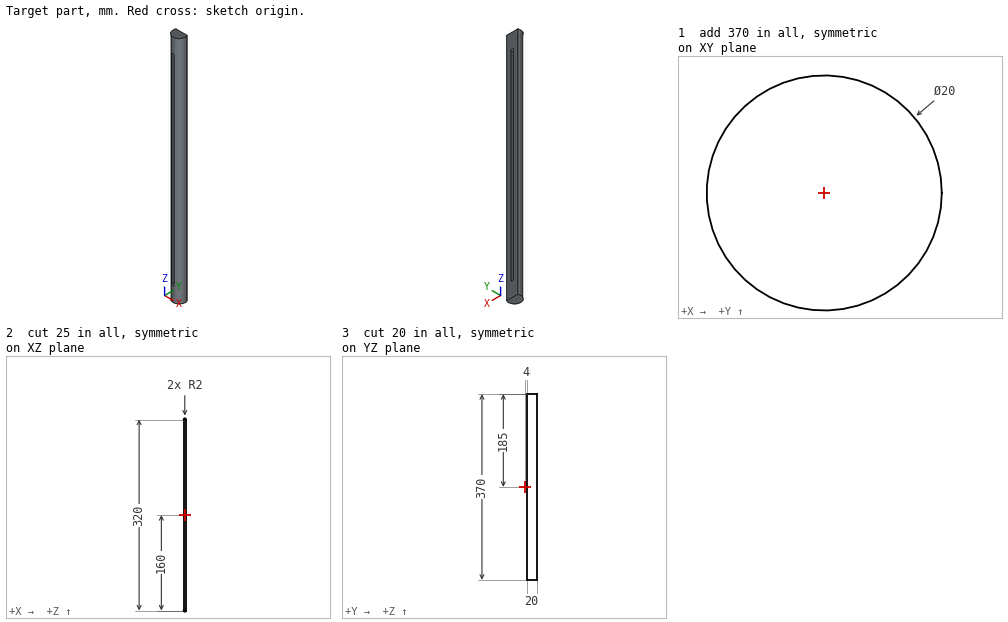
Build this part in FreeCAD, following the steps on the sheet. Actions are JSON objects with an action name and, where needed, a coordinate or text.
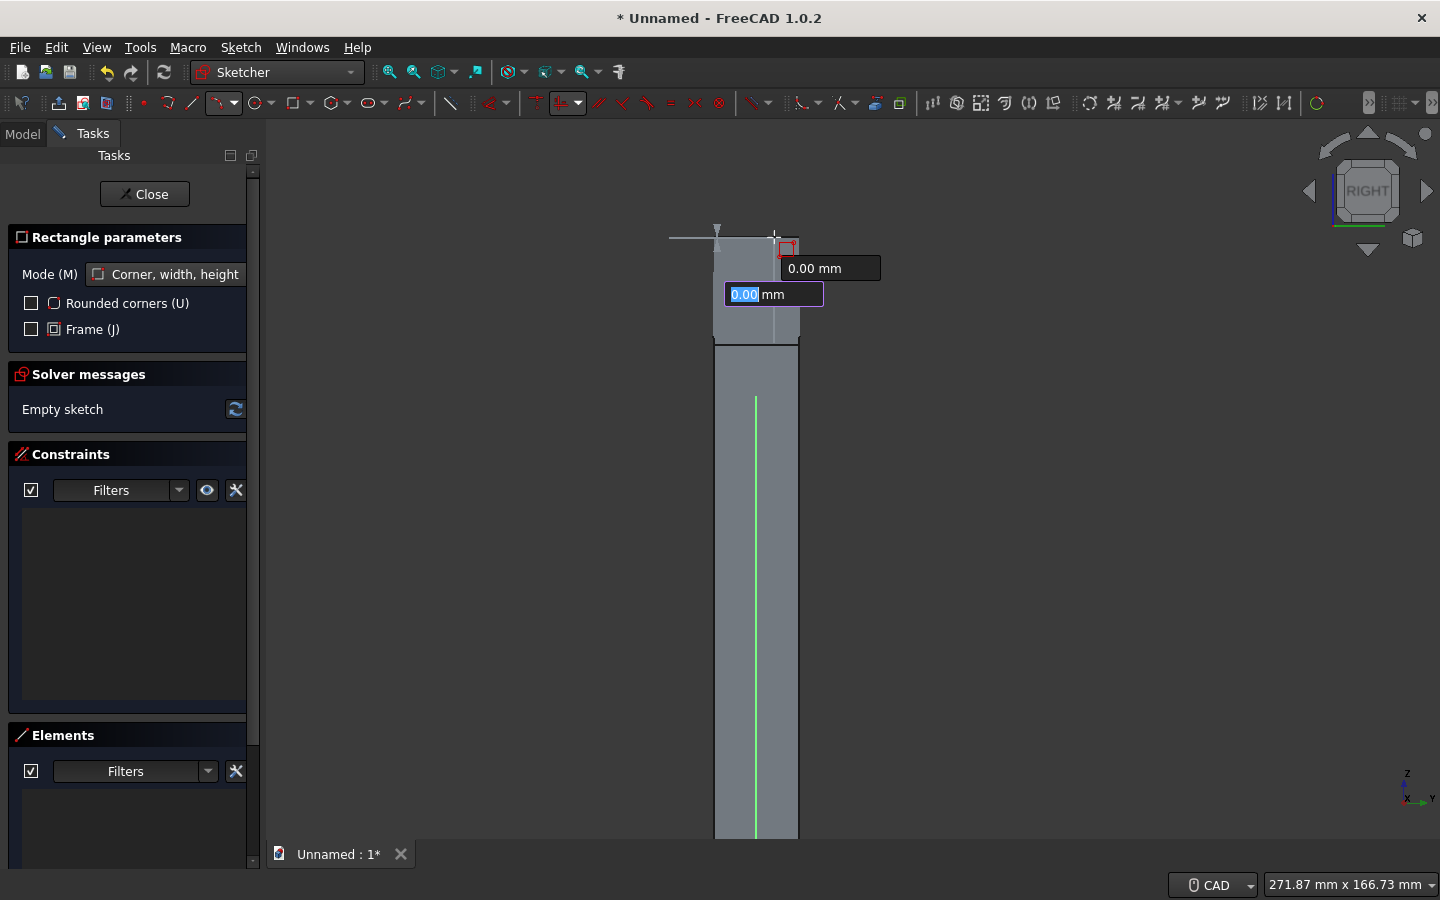
{"action": "scroll", "coordinate": [774, 239], "scroll_direction": "down", "scroll_amount": 6}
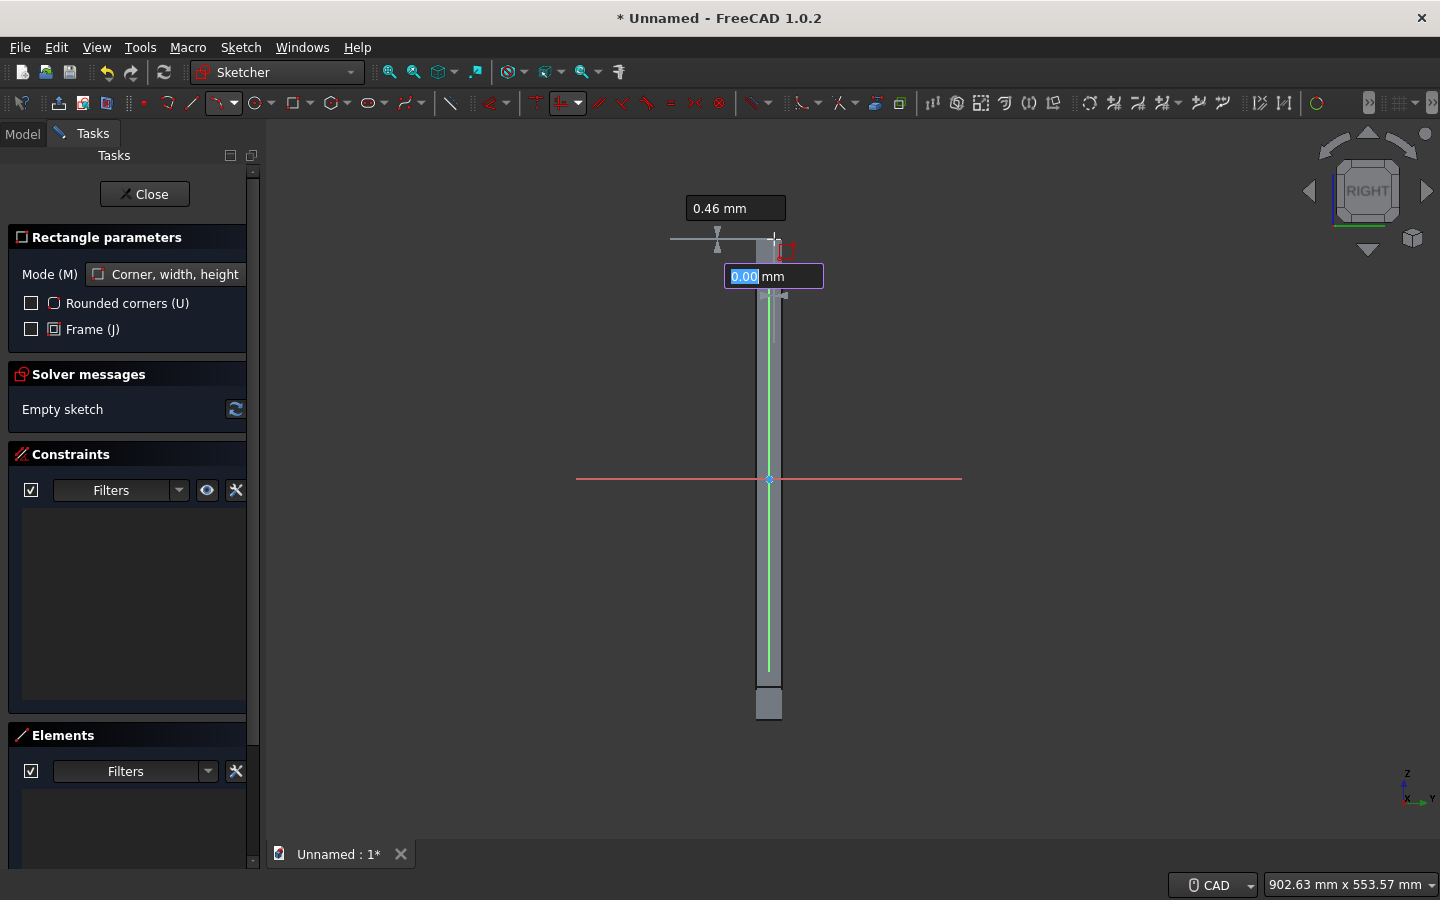
{"action": "left_click", "coordinate": [800, 720]}
{"action": "key", "text": "Escape"}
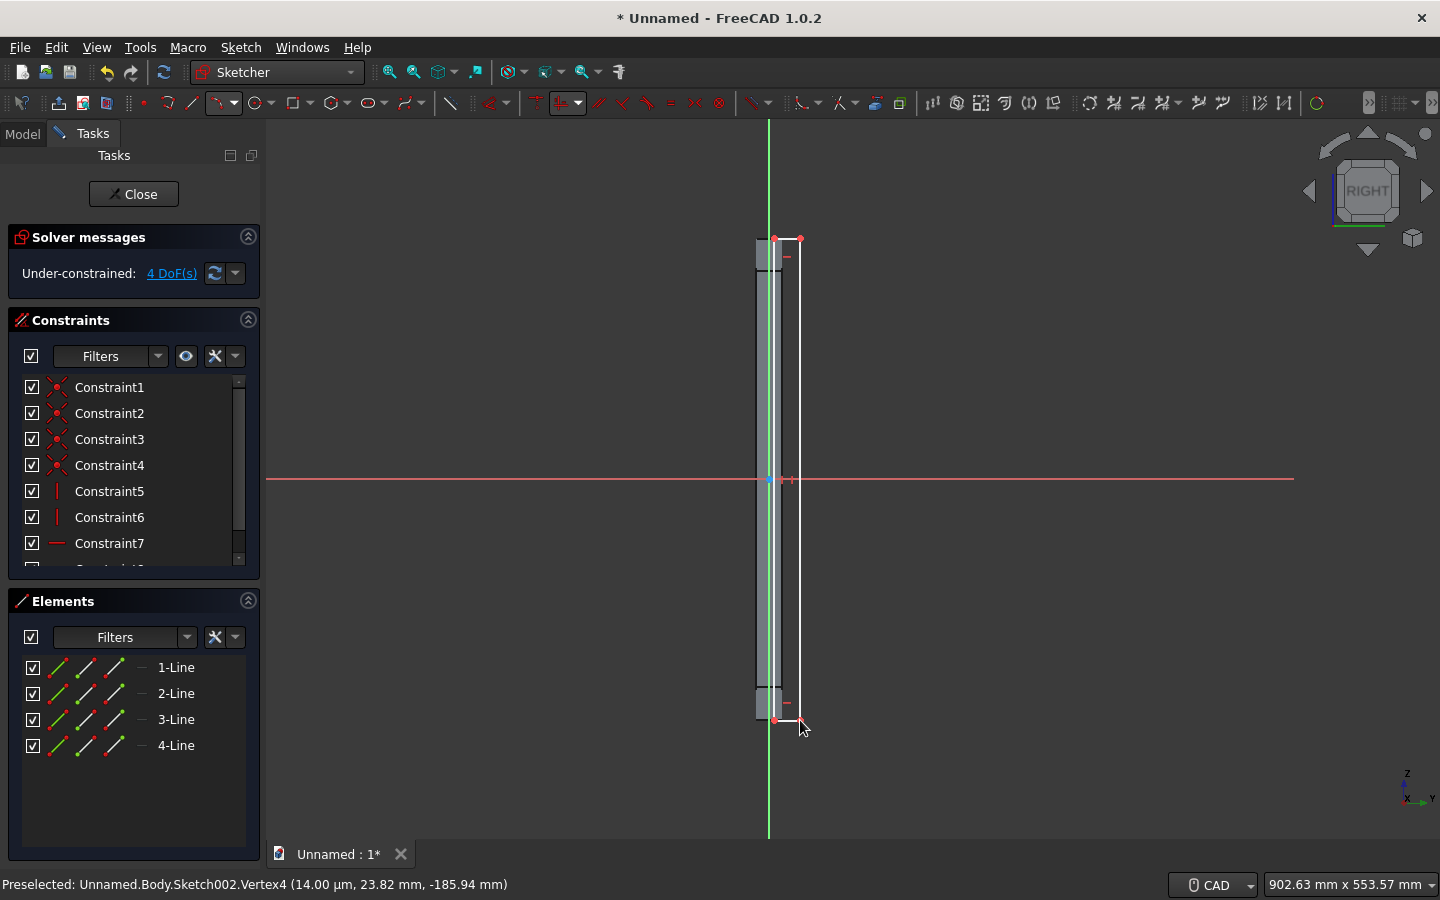
{"action": "left_click", "coordinate": [490, 104]}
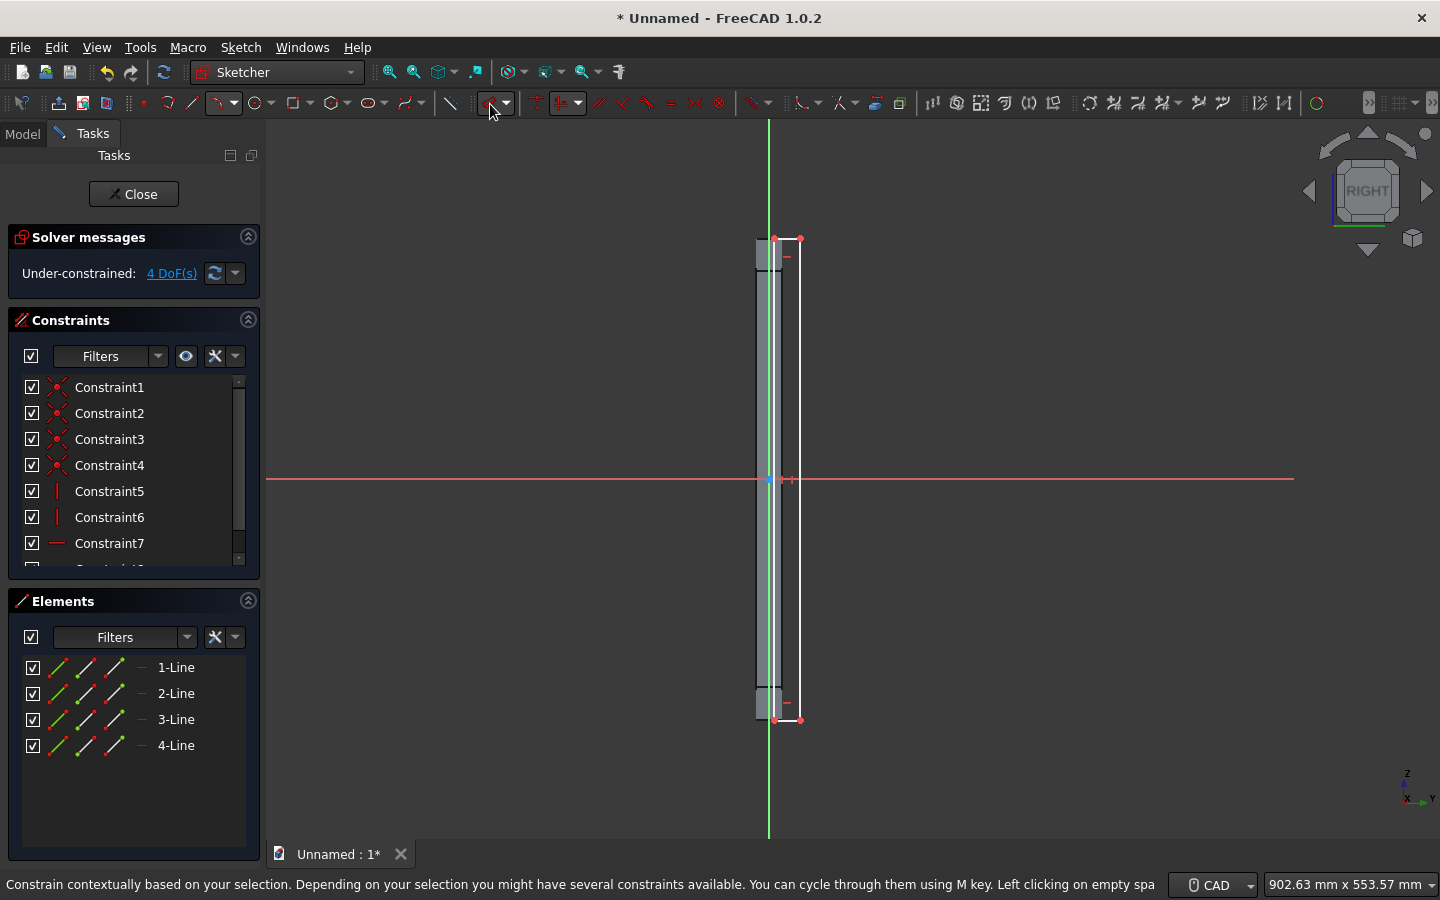
{"action": "scroll", "coordinate": [785, 721], "scroll_direction": "up", "scroll_amount": 3}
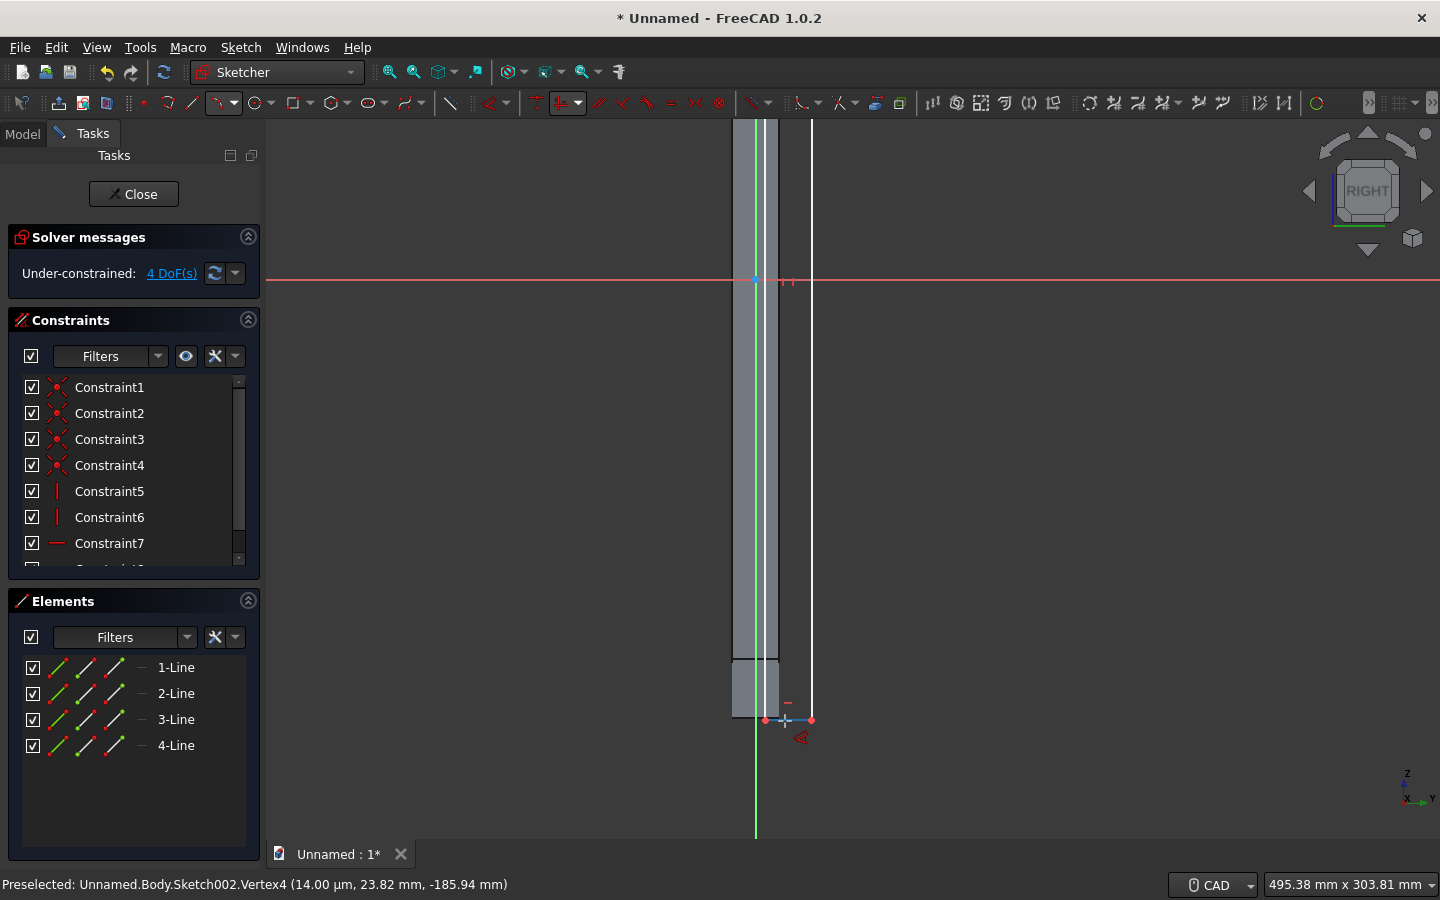
{"action": "left_click", "coordinate": [784, 720]}
{"action": "left_click", "coordinate": [789, 754]}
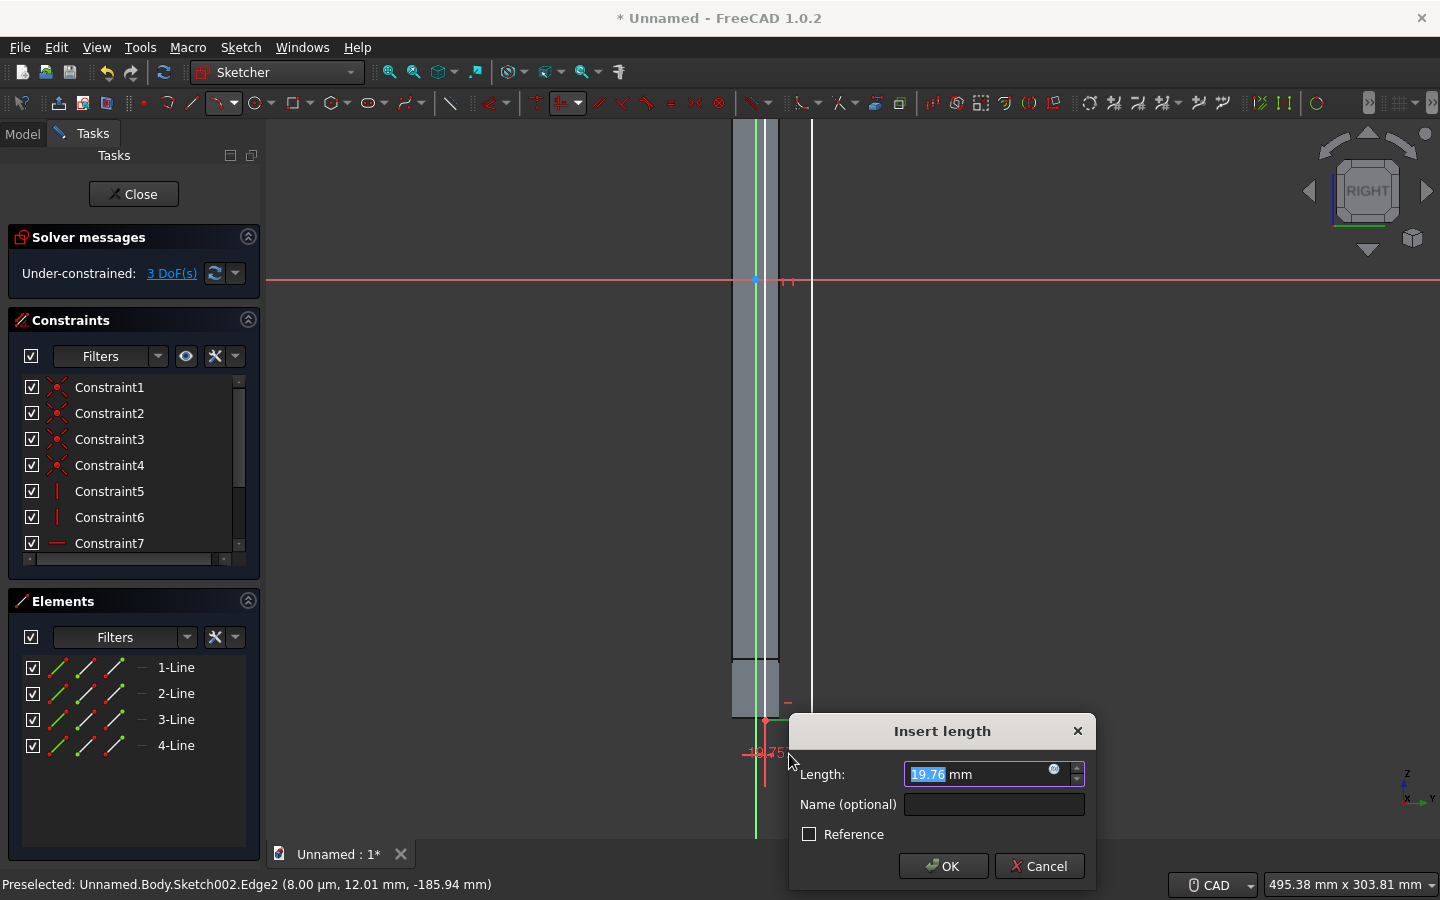
{"action": "type", "text": "20"}
{"action": "key", "text": "Return"}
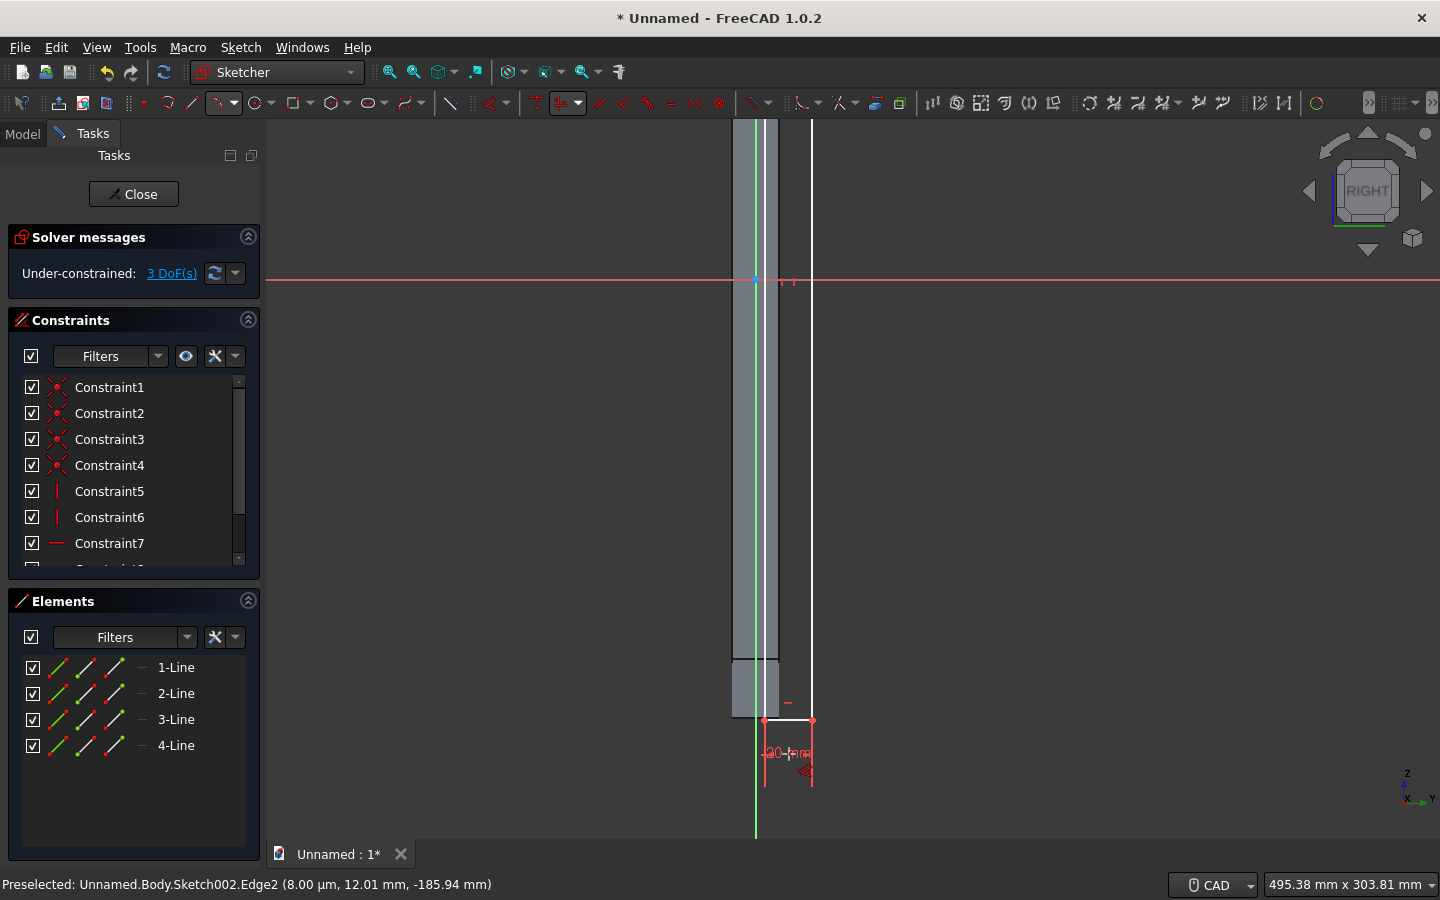
{"action": "scroll", "coordinate": [785, 721], "scroll_direction": "down", "scroll_amount": 3}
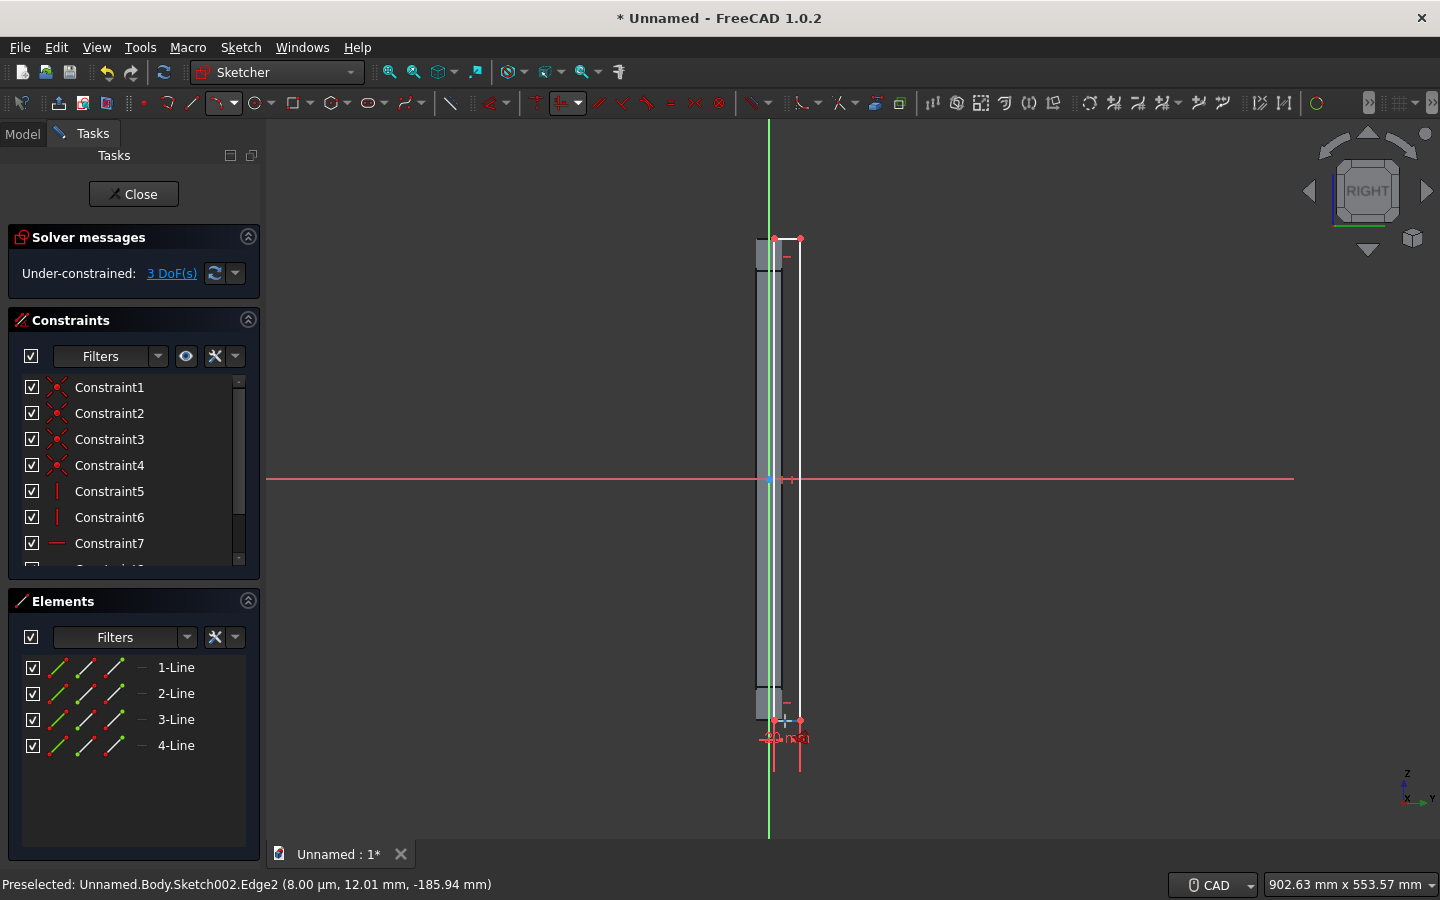
{"action": "scroll", "coordinate": [774, 239], "scroll_direction": "up", "scroll_amount": 11}